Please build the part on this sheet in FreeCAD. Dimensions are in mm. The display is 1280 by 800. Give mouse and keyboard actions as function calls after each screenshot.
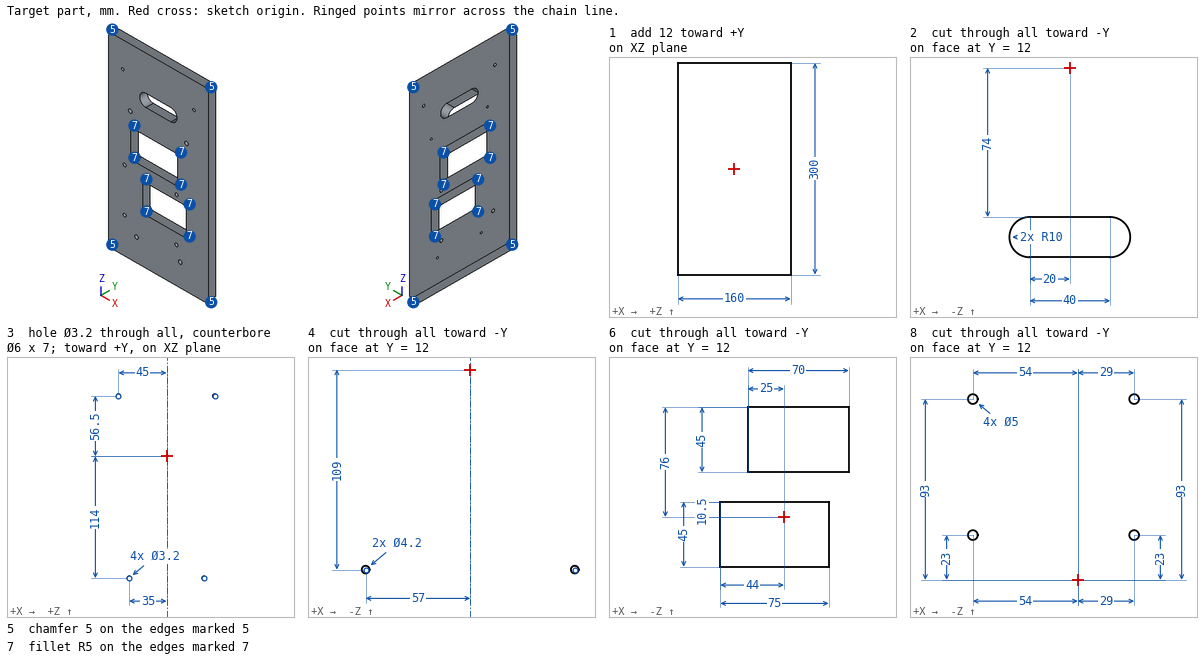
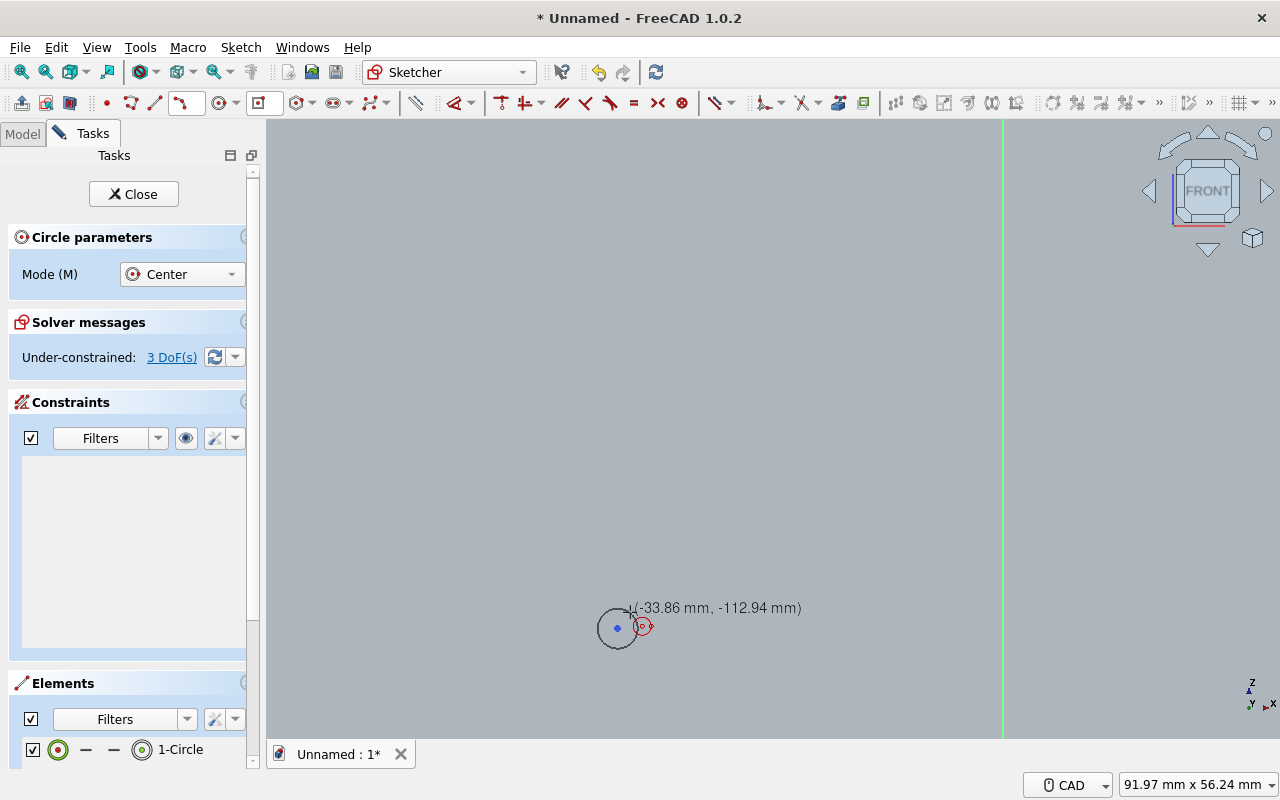
scroll(629, 617, down, 8)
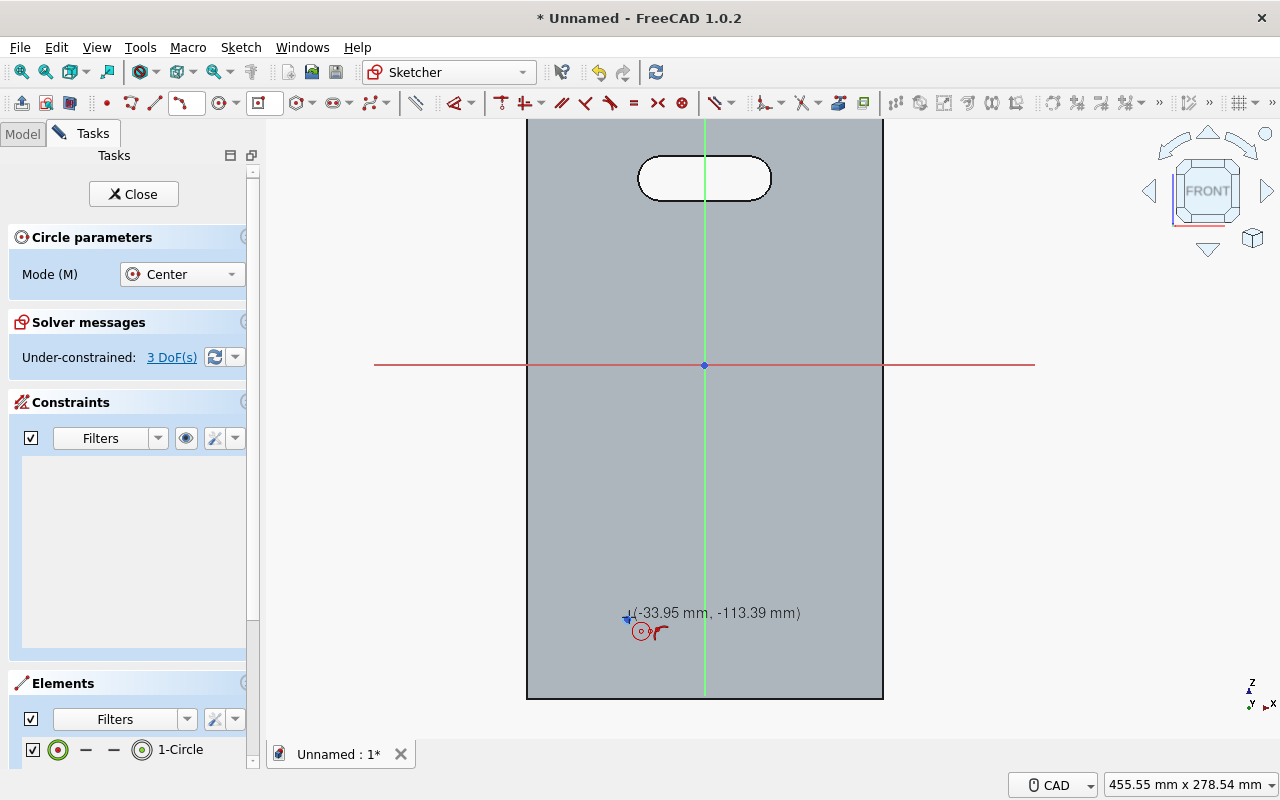
scroll(783, 619, up, 10)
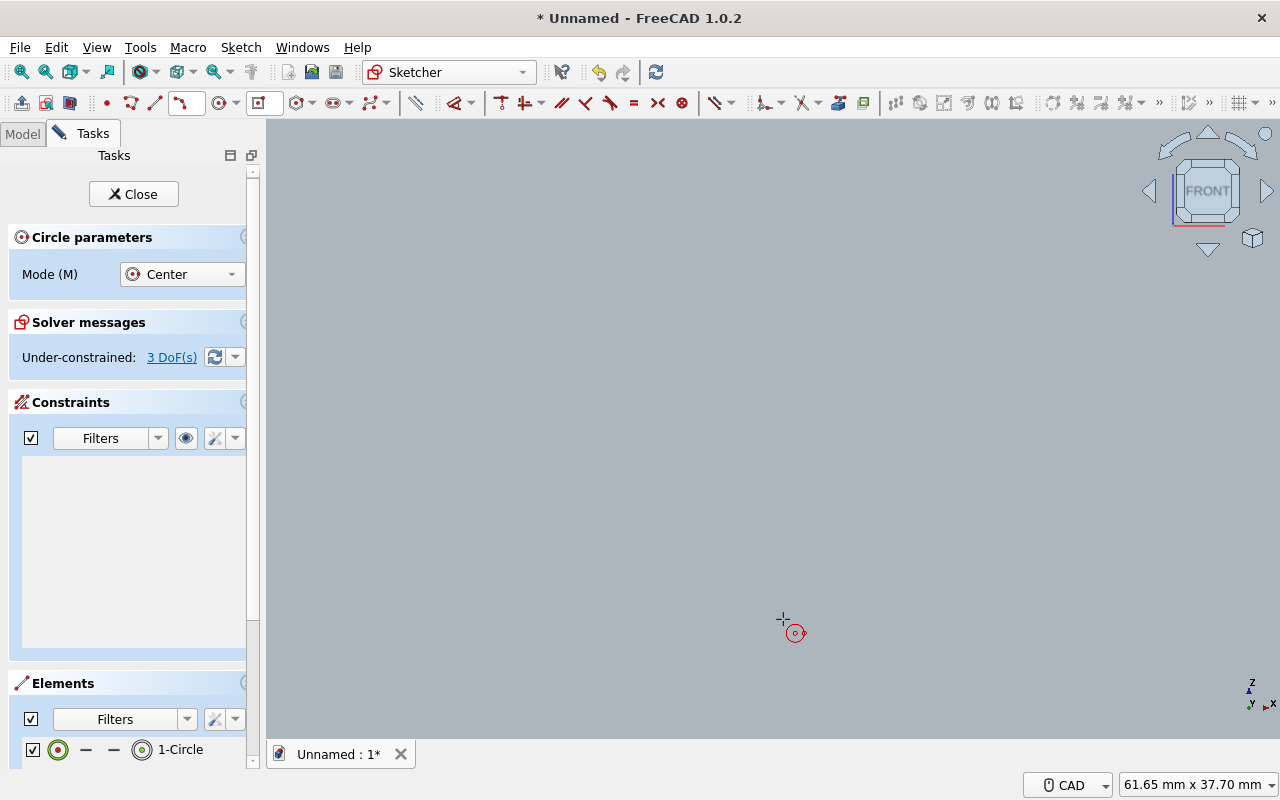
scroll(783, 619, down, 10)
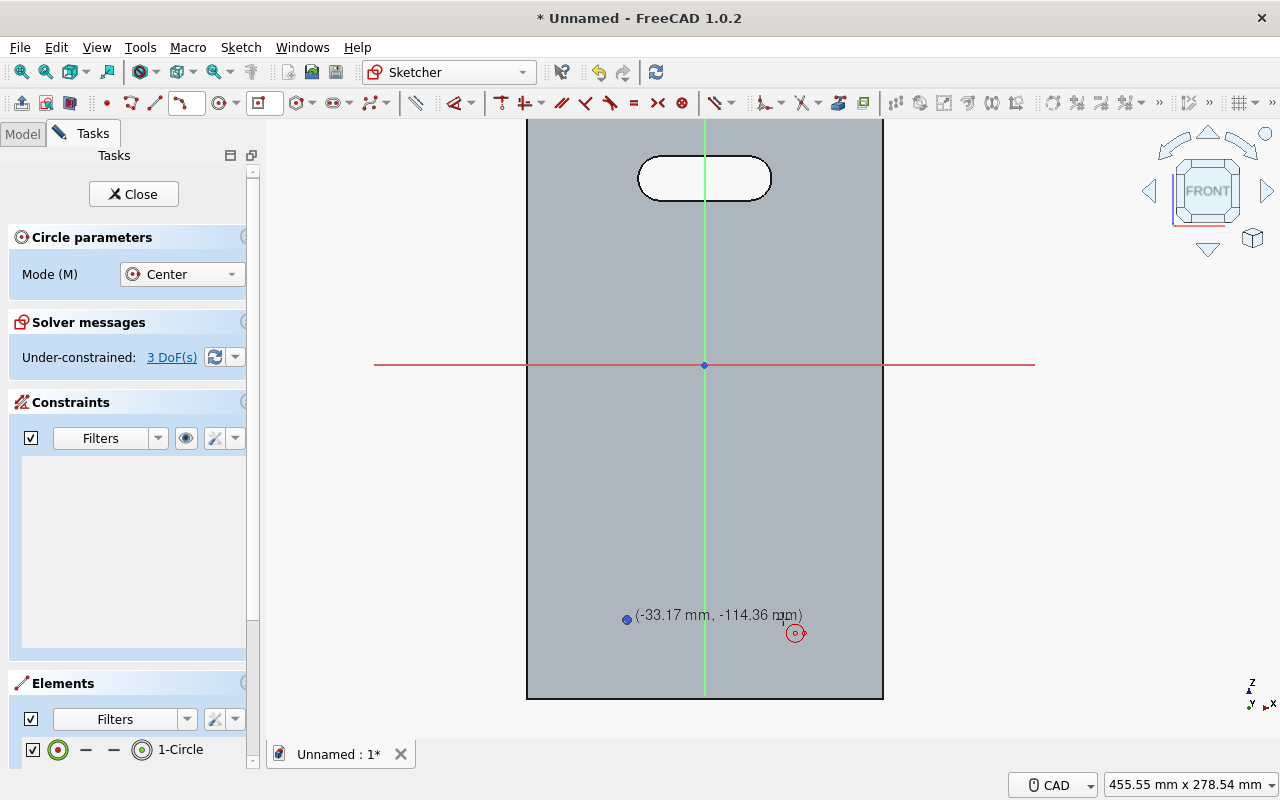
click(783, 619)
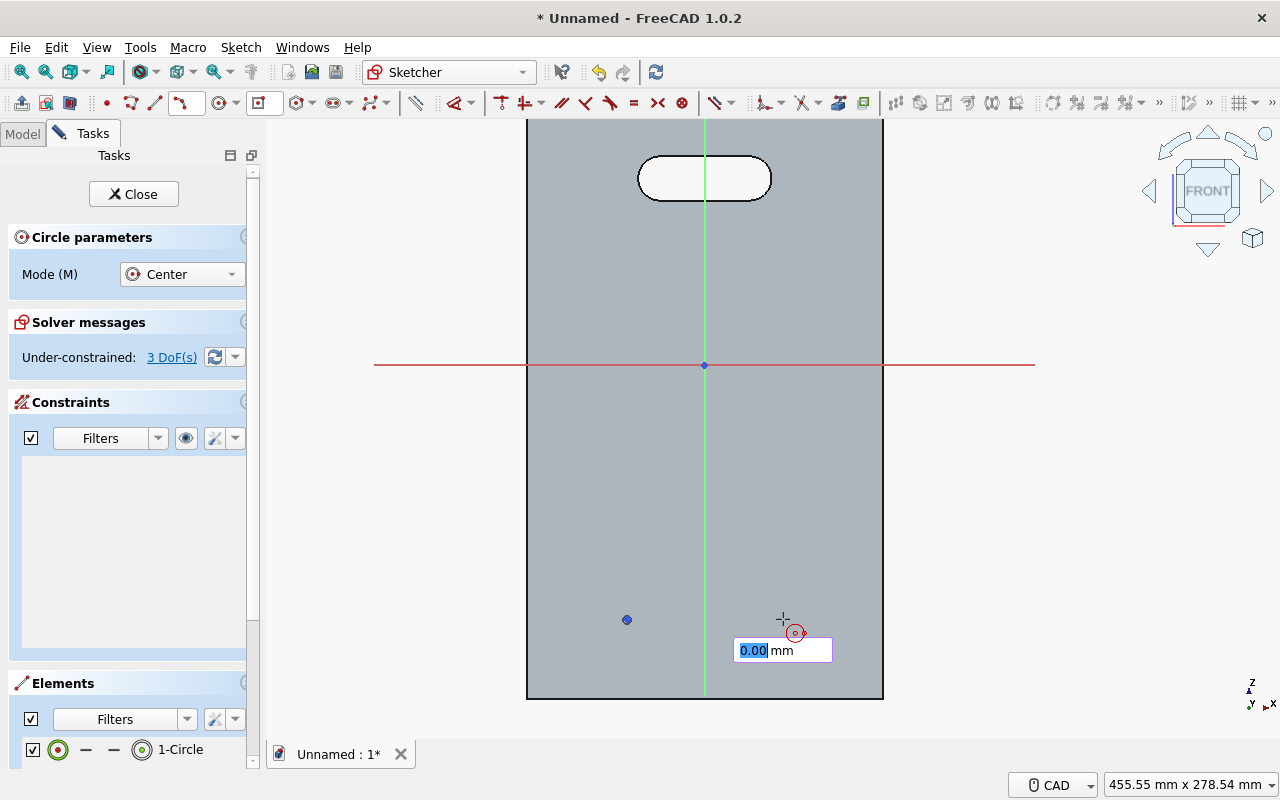
scroll(785, 617, up, 8)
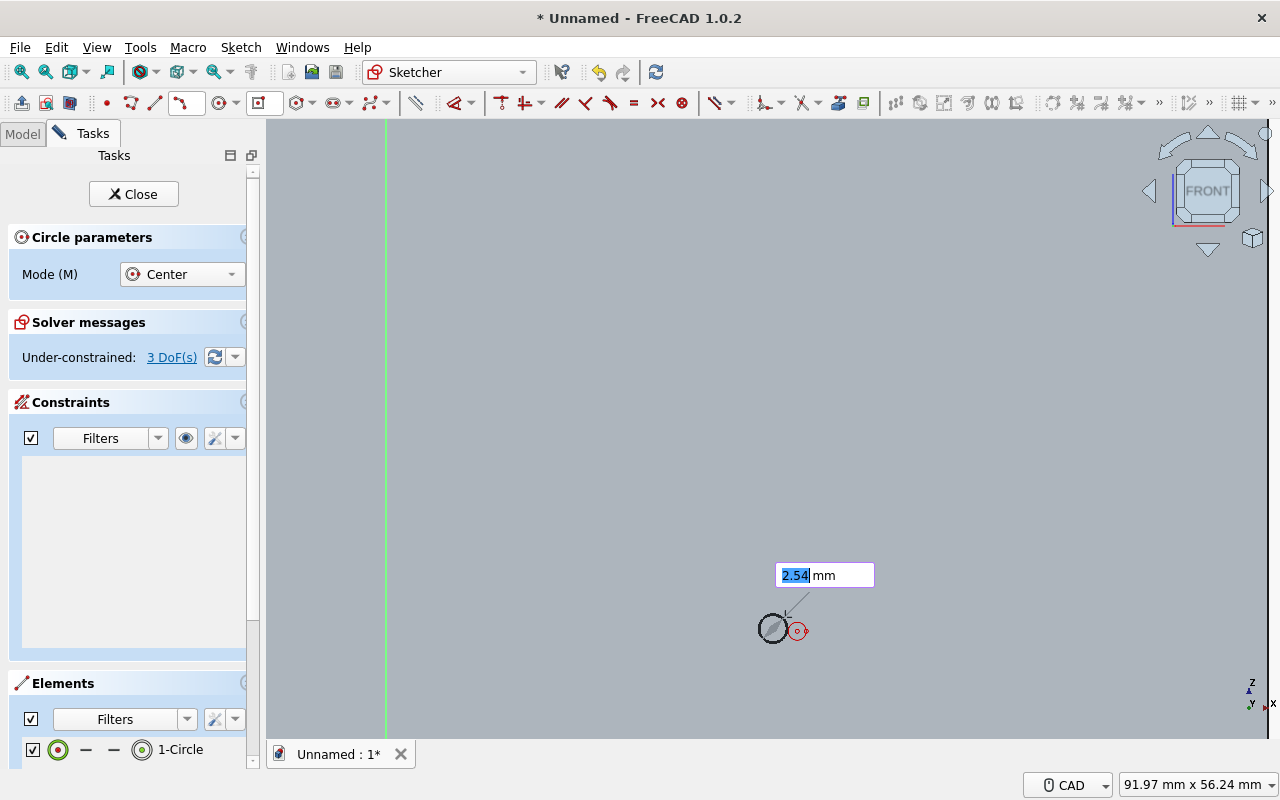
click(784, 612)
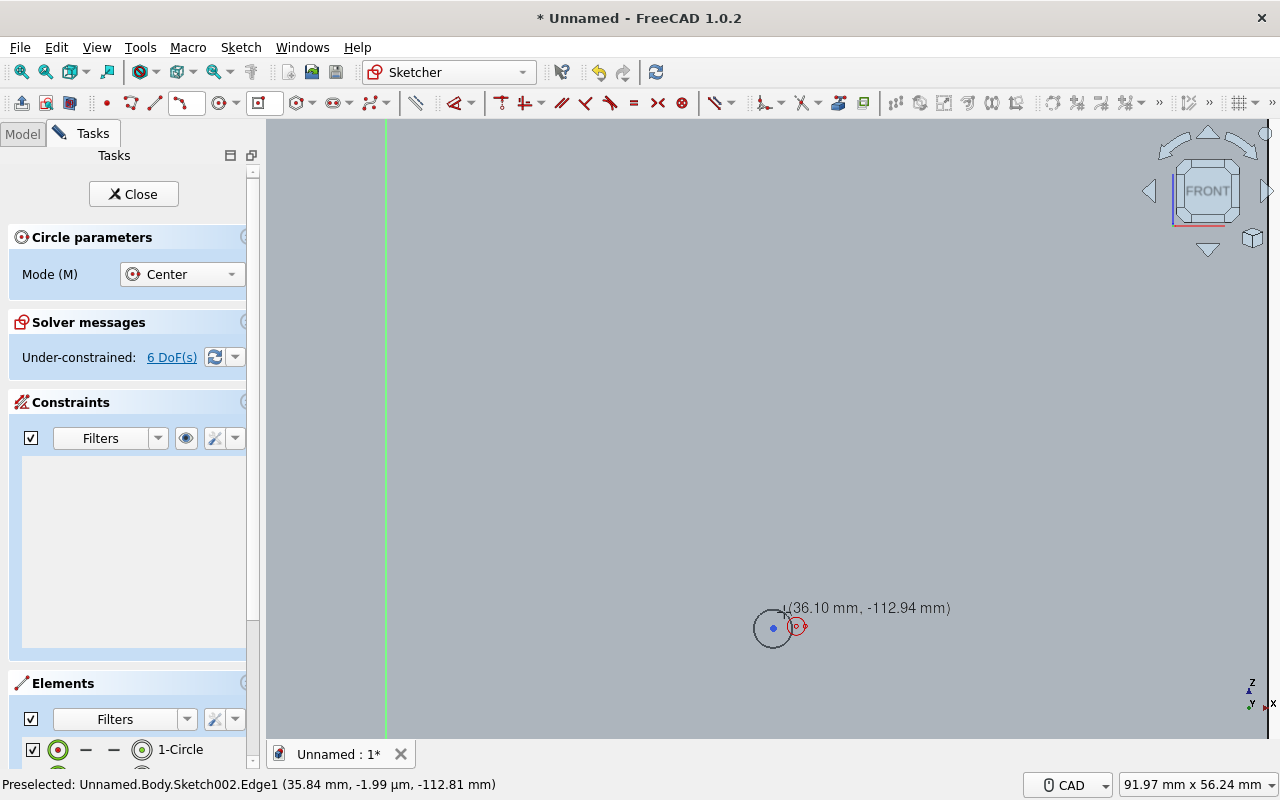
scroll(785, 617, down, 8)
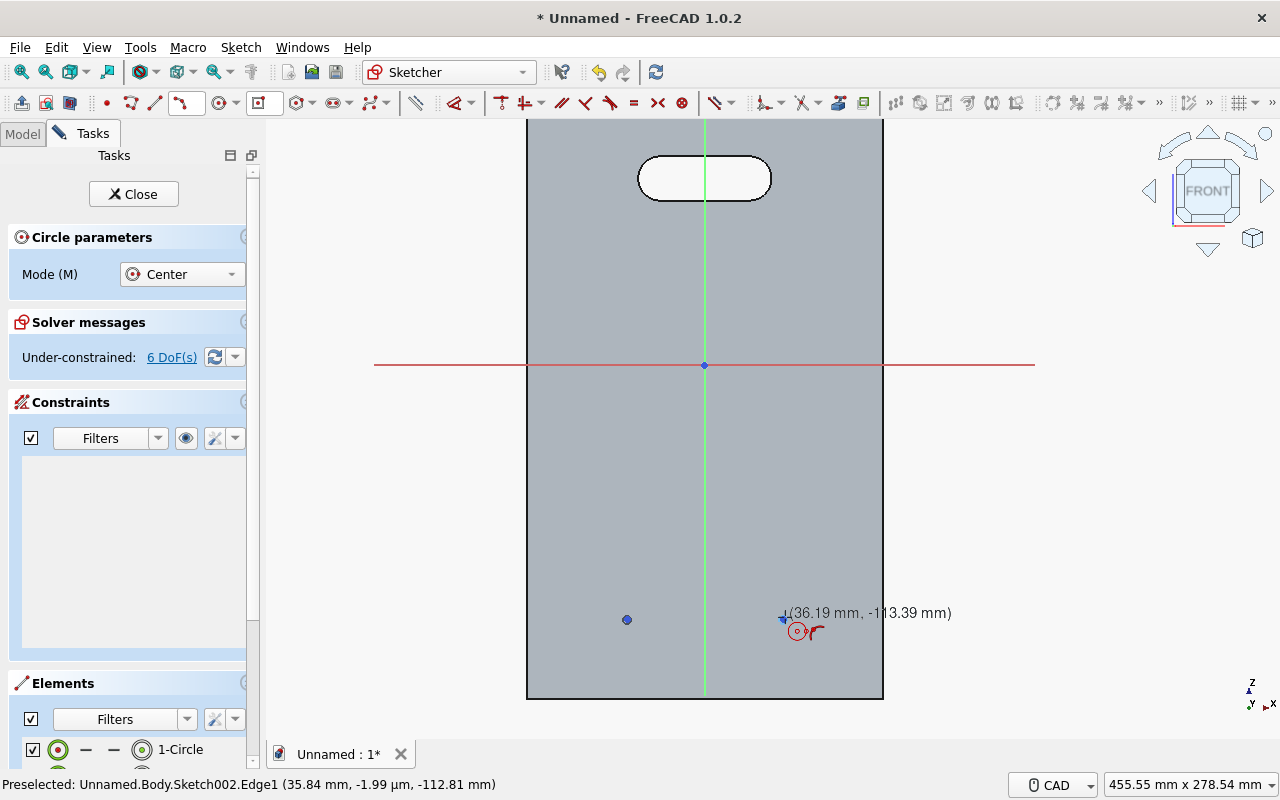
scroll(605, 240, up, 10)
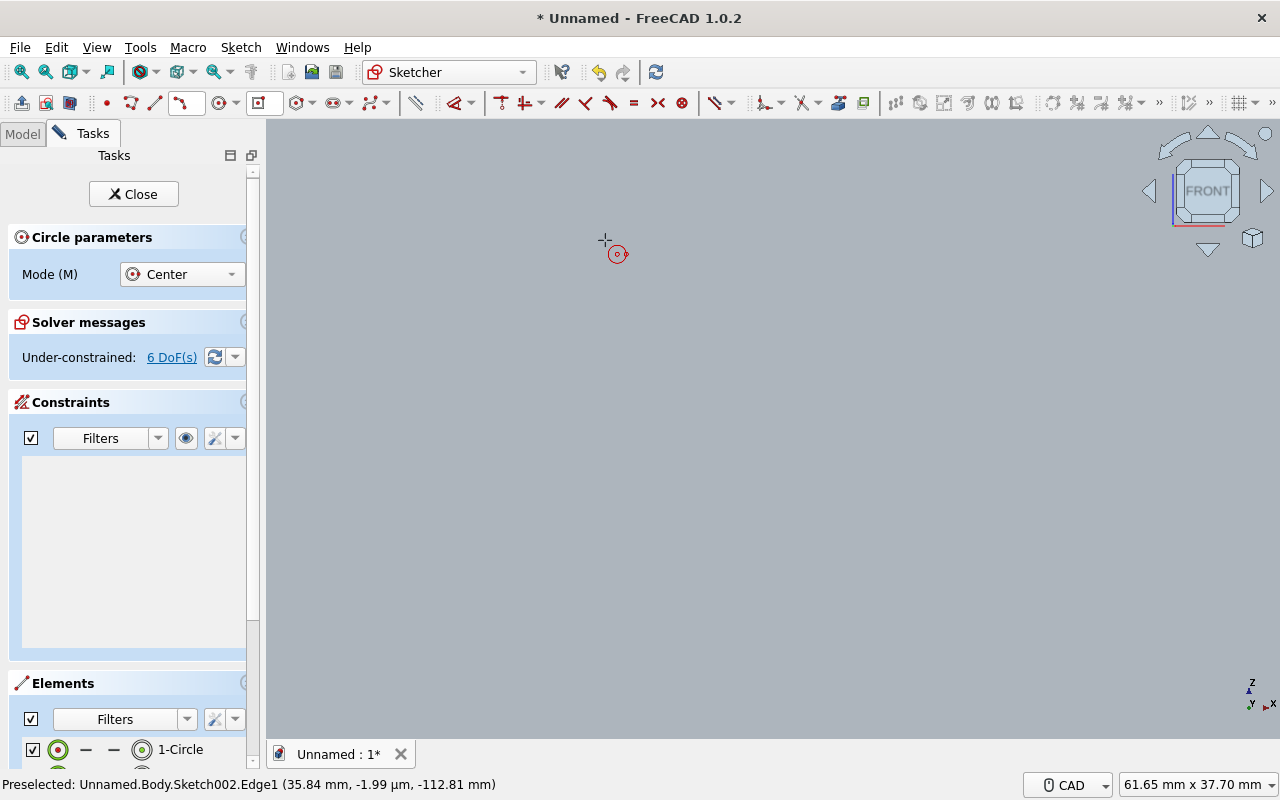
scroll(605, 240, down, 10)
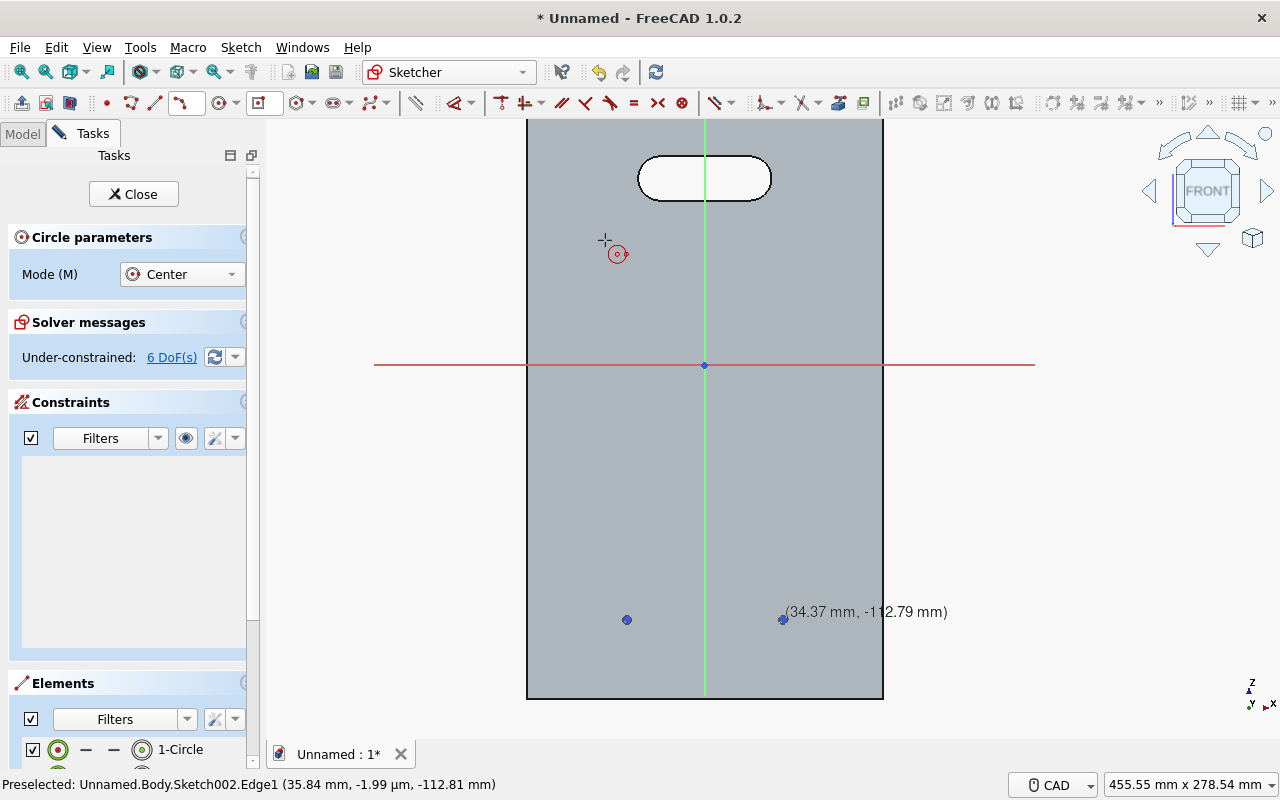
click(605, 240)